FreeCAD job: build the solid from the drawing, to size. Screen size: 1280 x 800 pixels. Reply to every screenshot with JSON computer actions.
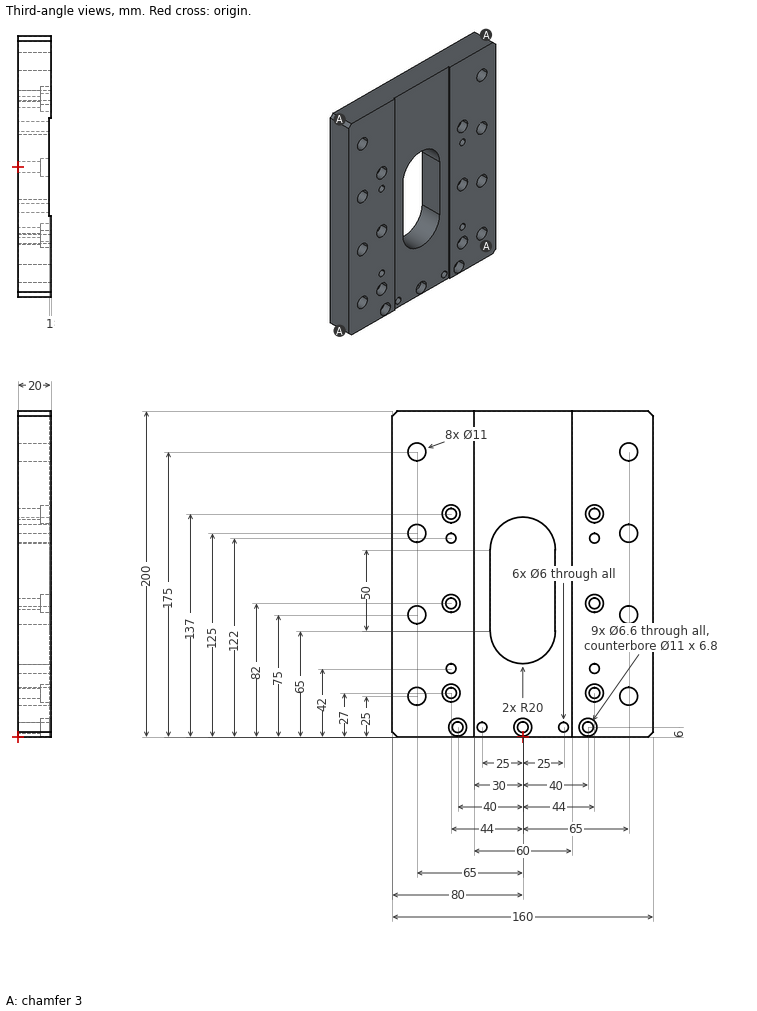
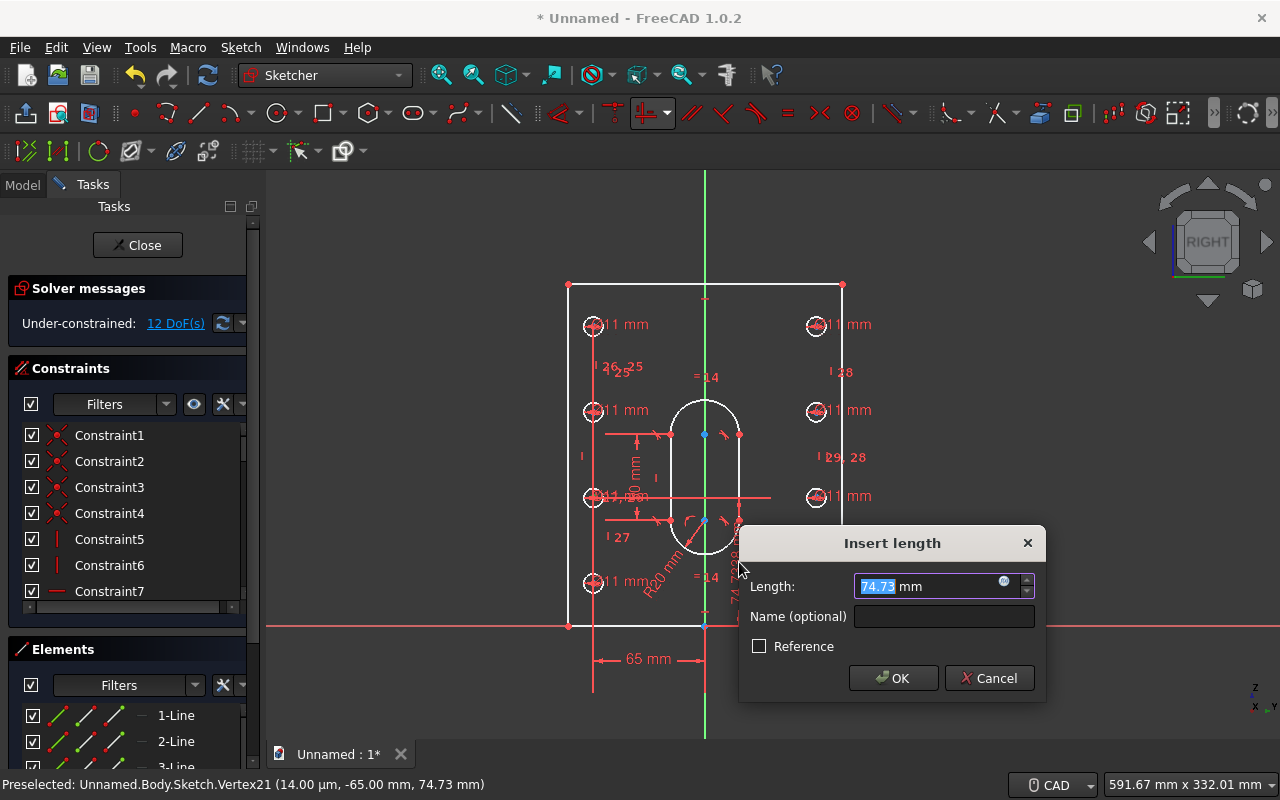
{"action": "type", "text": "75"}
{"action": "key", "text": "Return"}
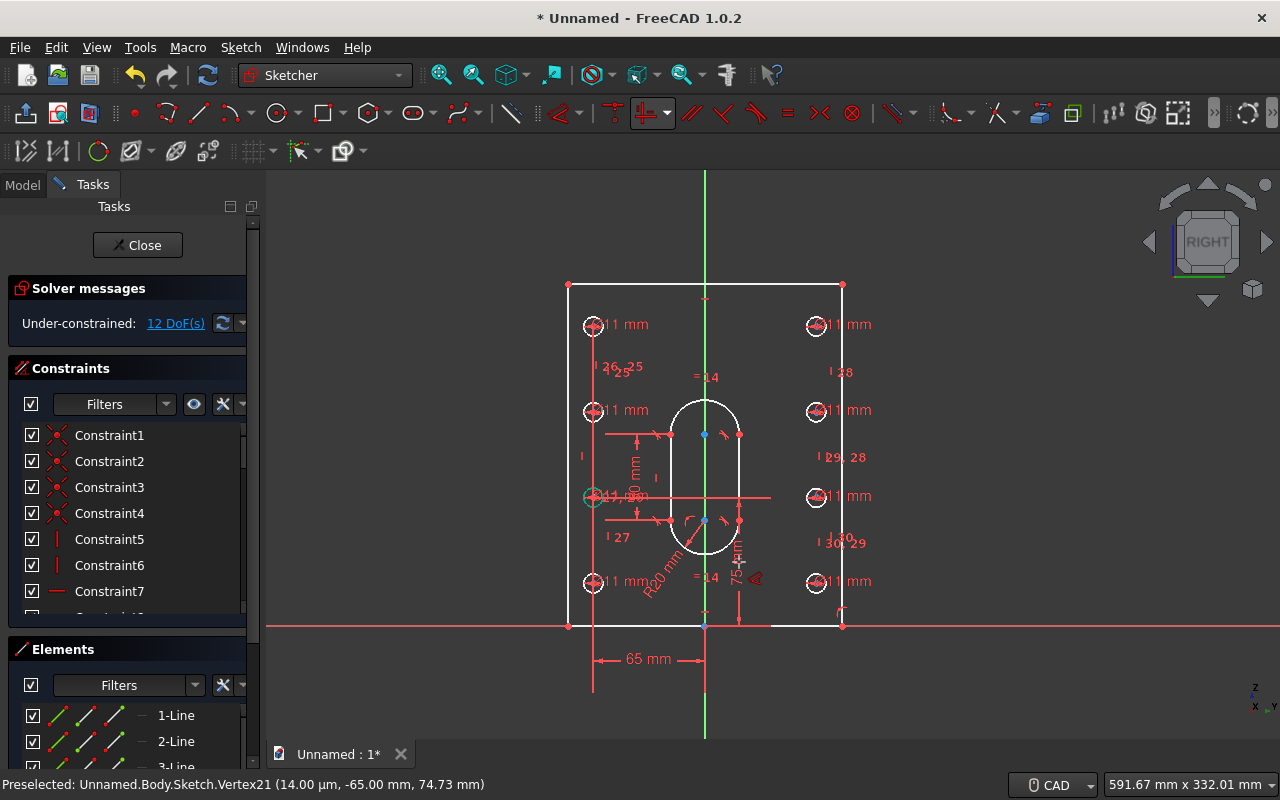
{"action": "left_click", "coordinate": [593, 583]}
{"action": "left_click", "coordinate": [739, 605]}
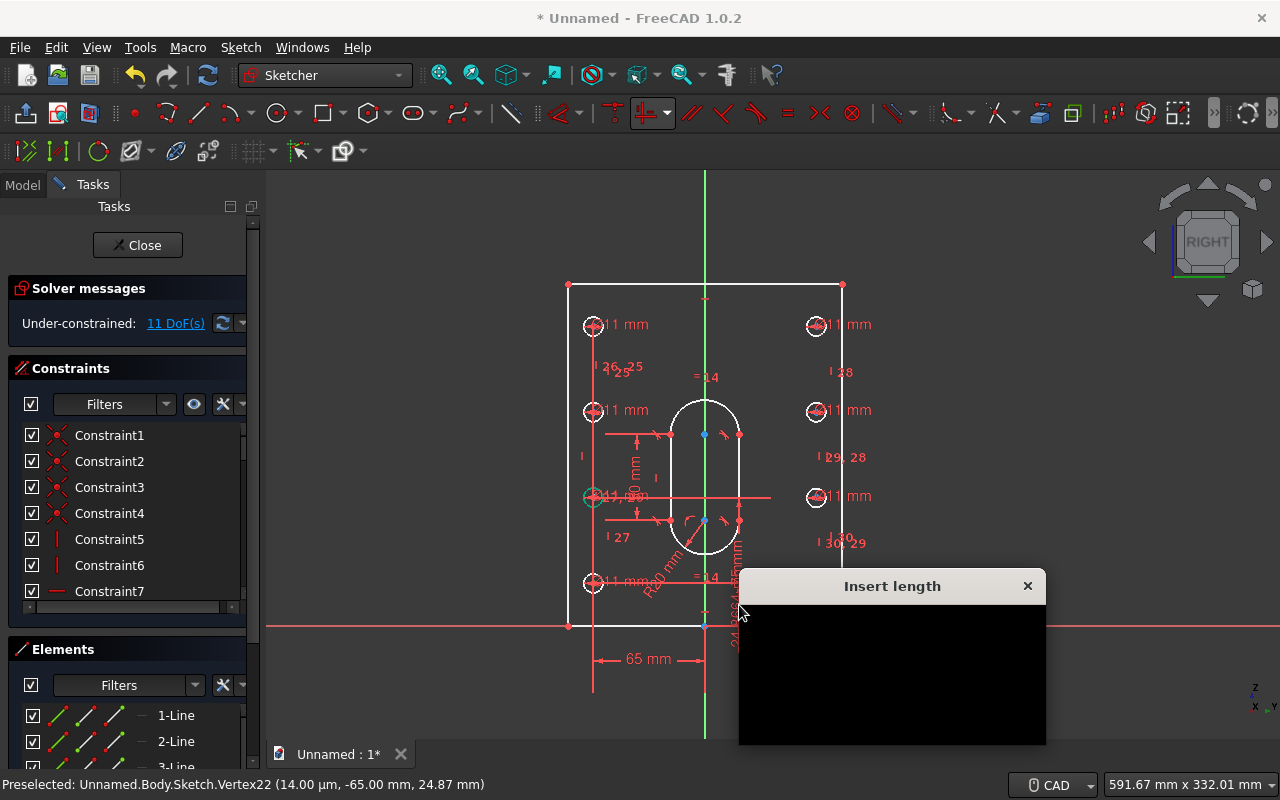
{"action": "type", "text": "25"}
{"action": "key", "text": "Return"}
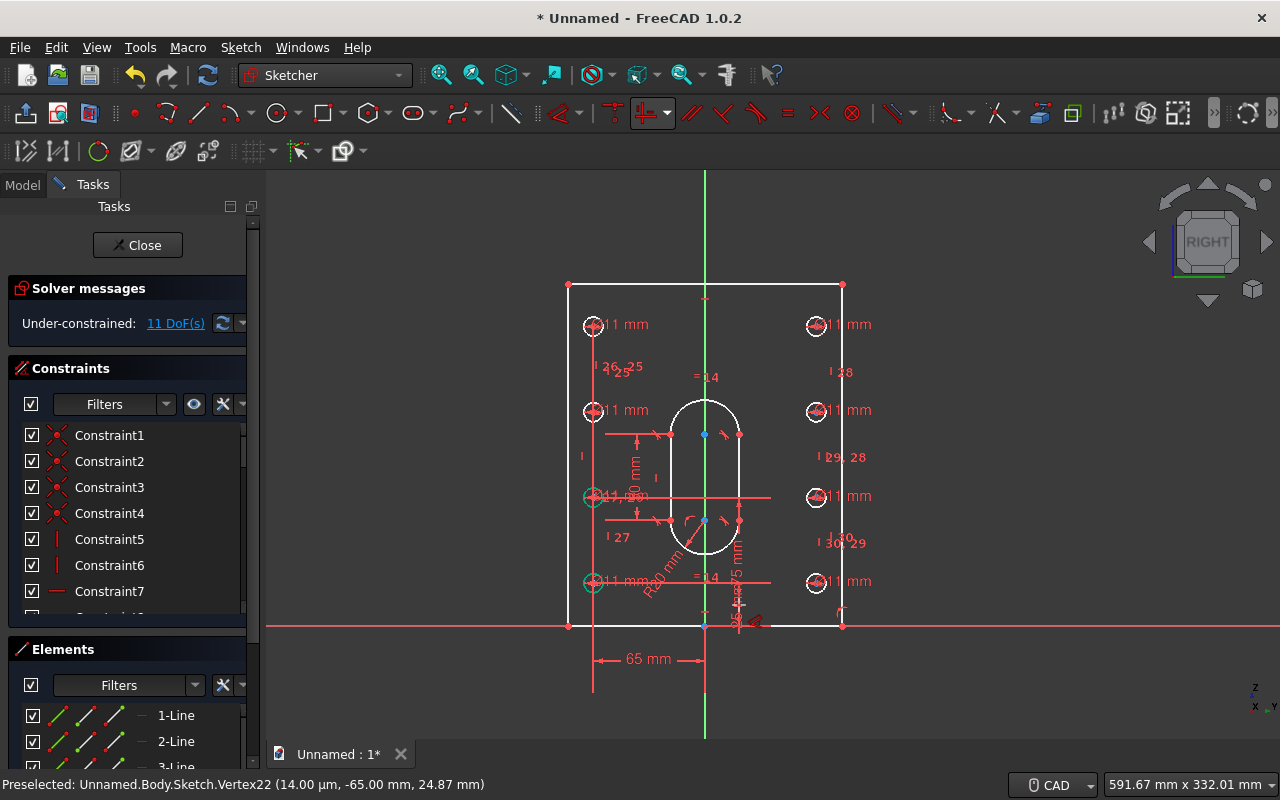
{"action": "left_click", "coordinate": [816, 327]}
{"action": "left_click", "coordinate": [761, 660]}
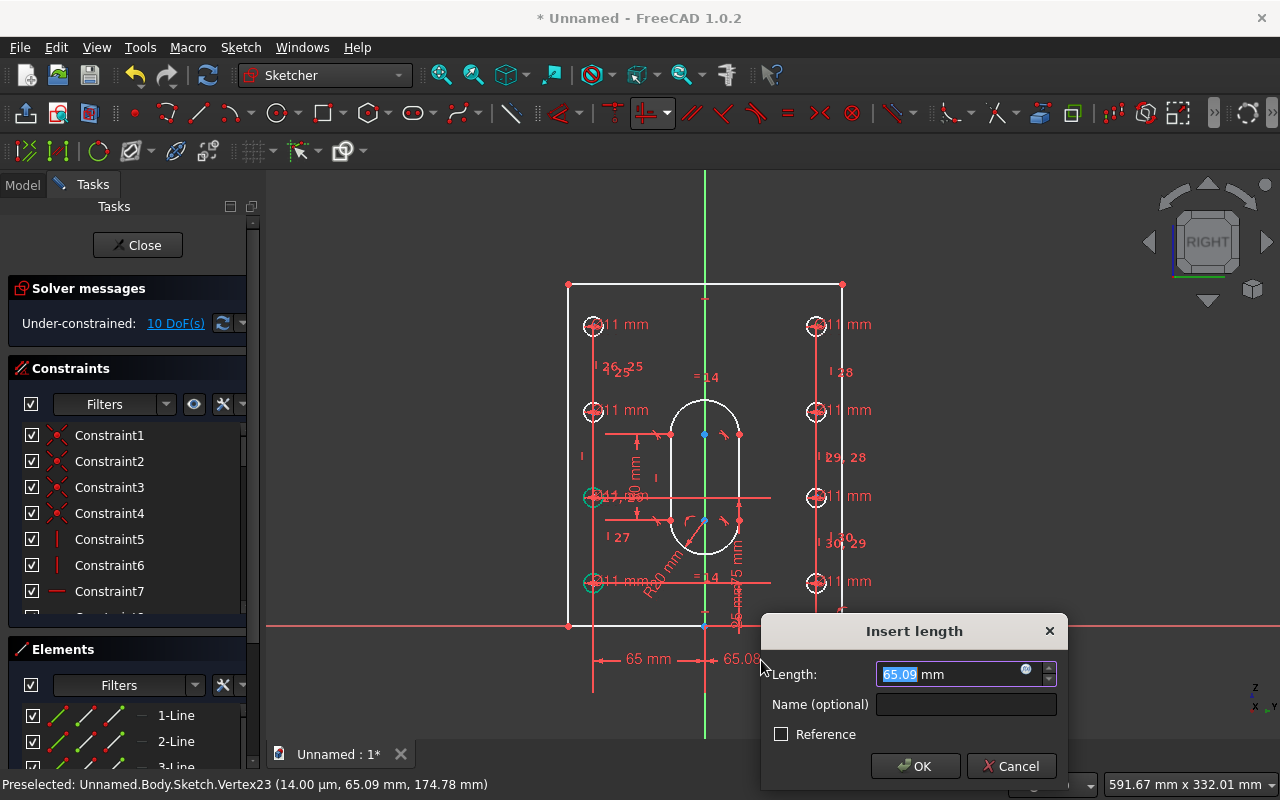
{"action": "type", "text": "65"}
{"action": "key", "text": "Return"}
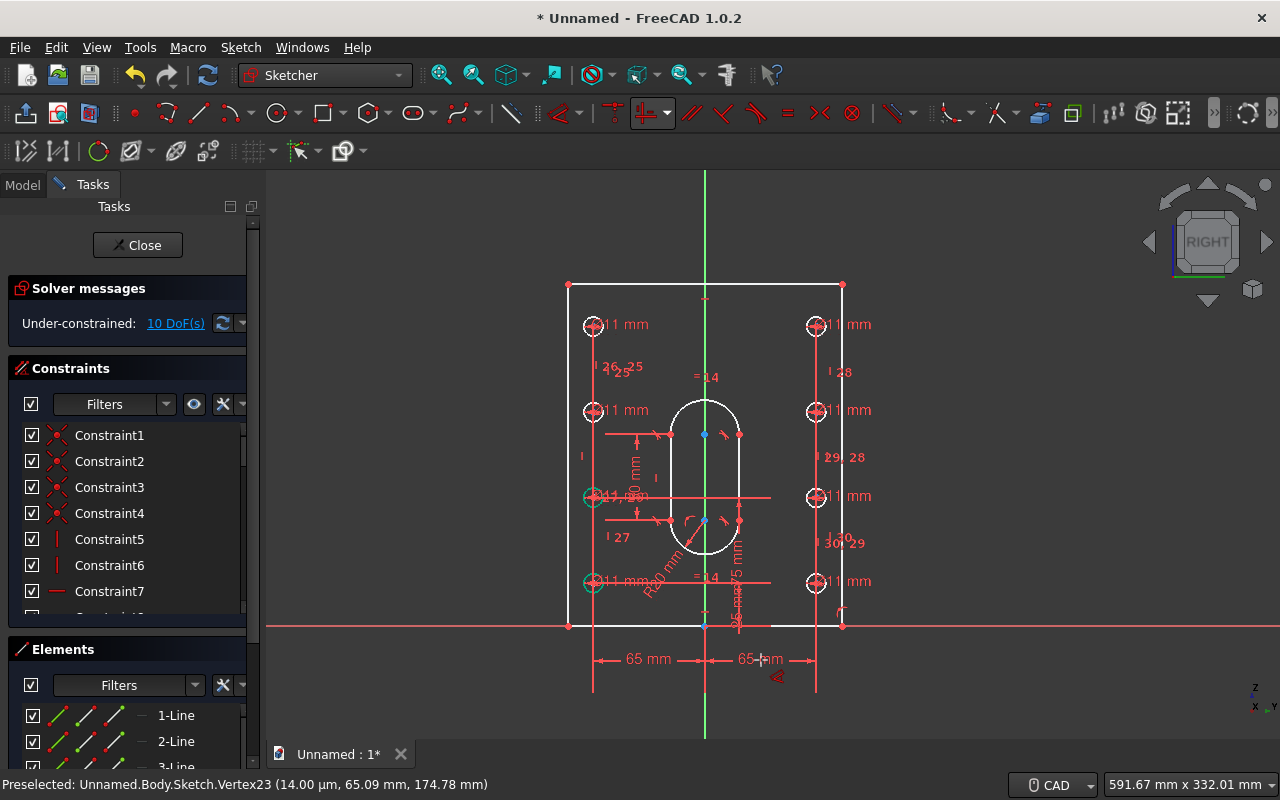
{"action": "left_click", "coordinate": [816, 498]}
{"action": "left_click", "coordinate": [874, 562]}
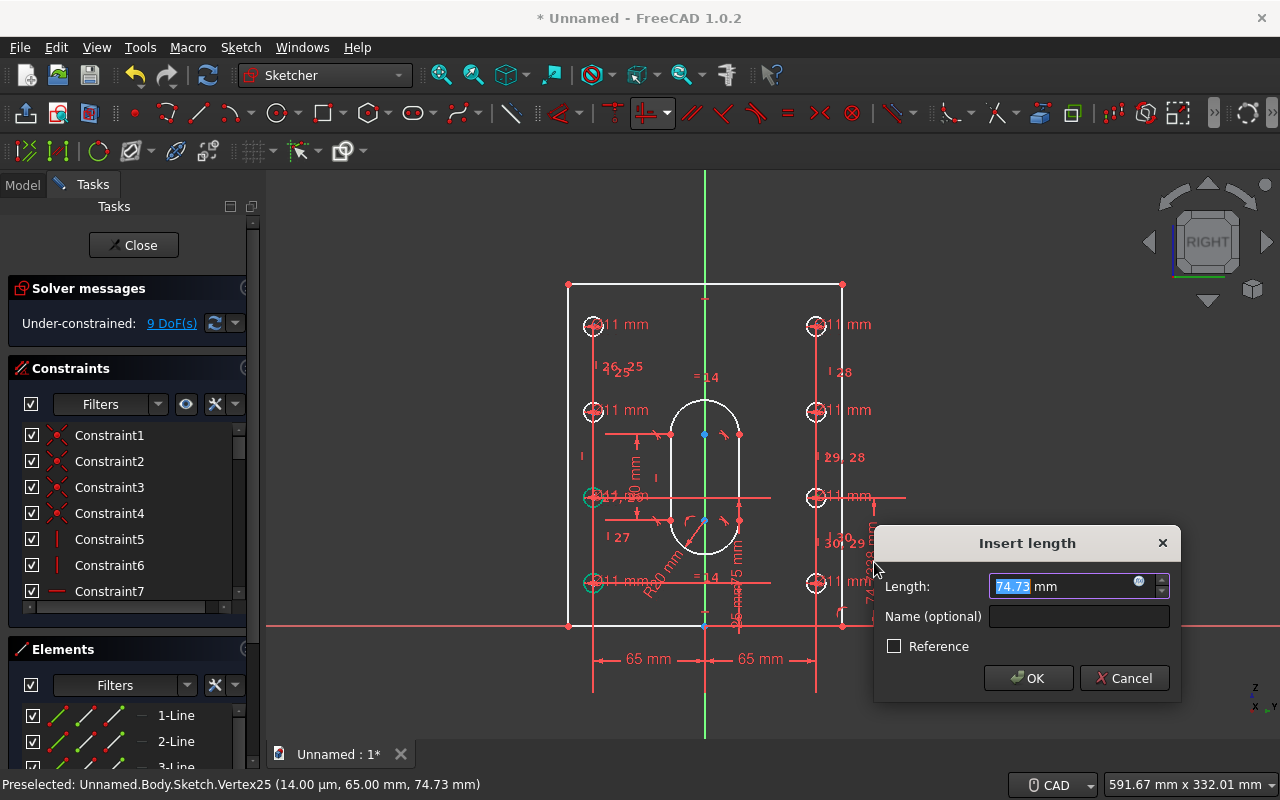
{"action": "type", "text": "75"}
{"action": "key", "text": "Return"}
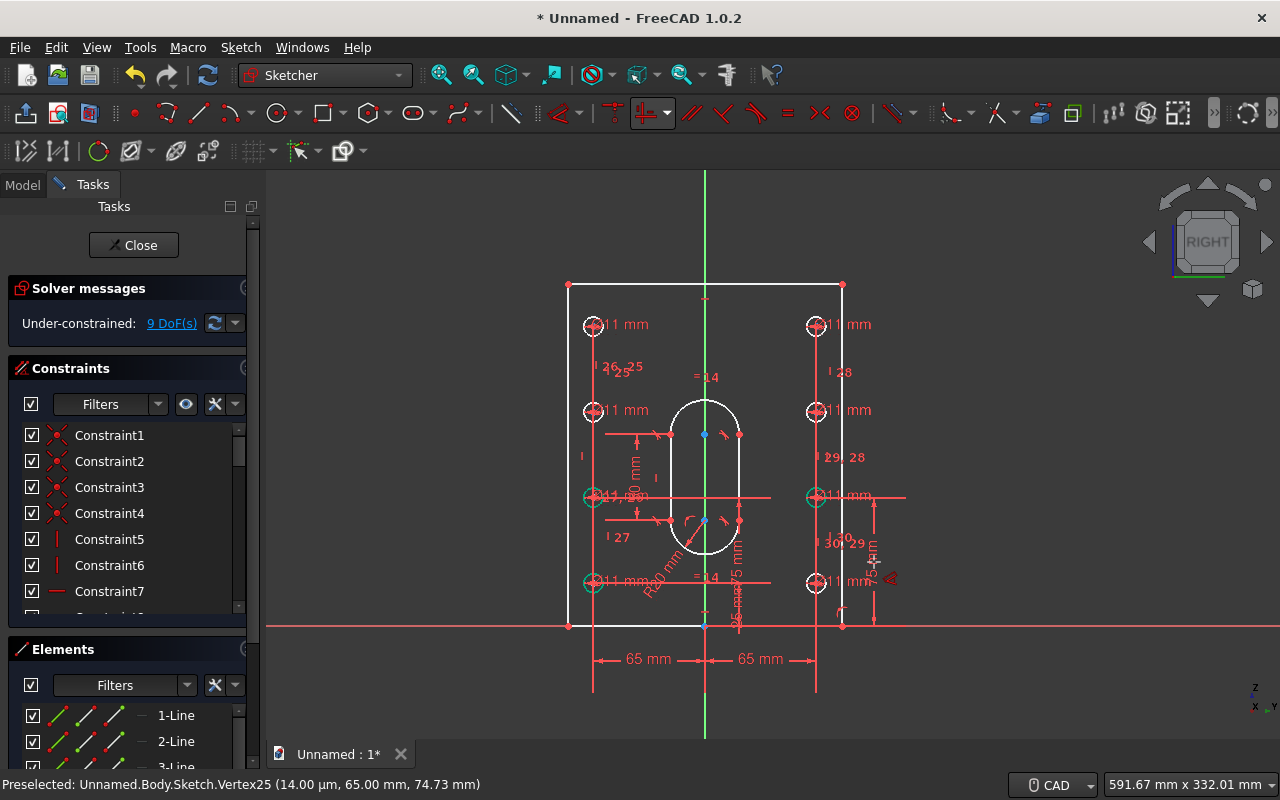
{"action": "left_click", "coordinate": [816, 583]}
{"action": "left_click", "coordinate": [874, 605]}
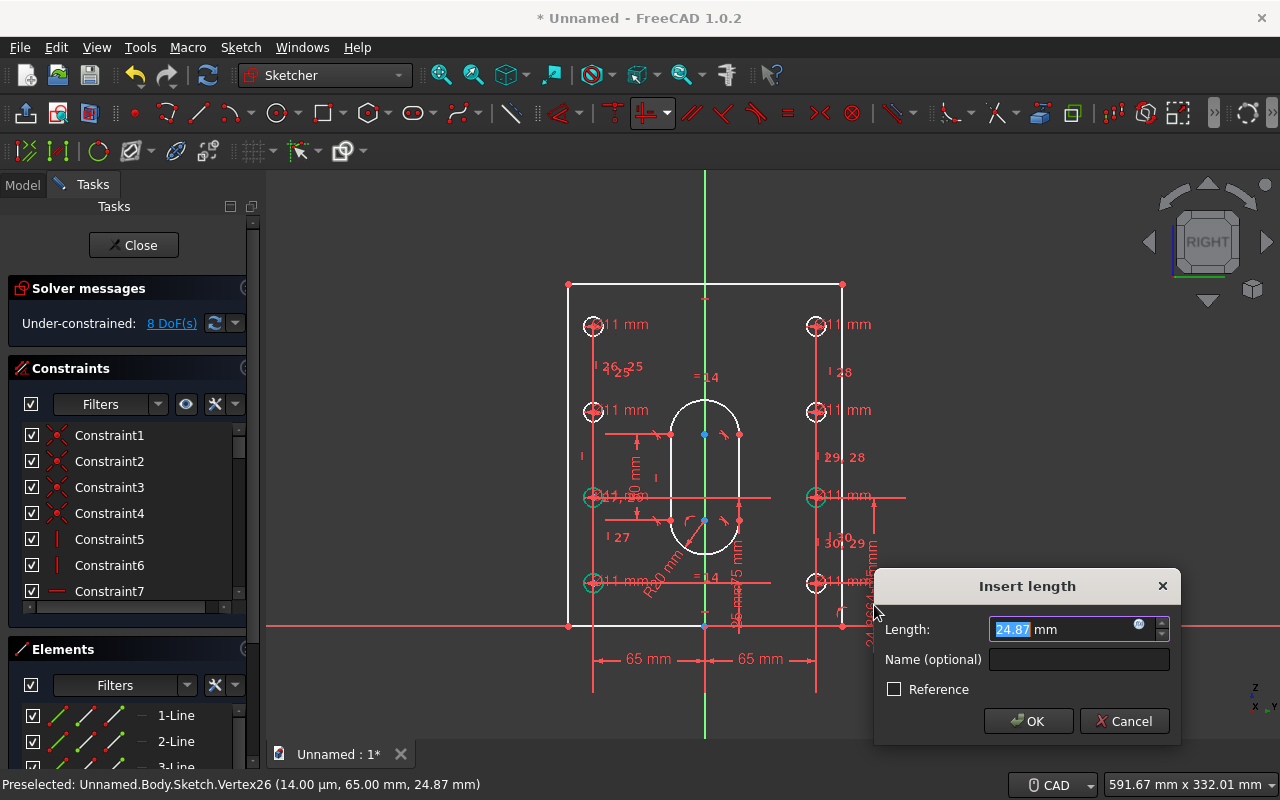
{"action": "type", "text": "25"}
{"action": "key", "text": "Return"}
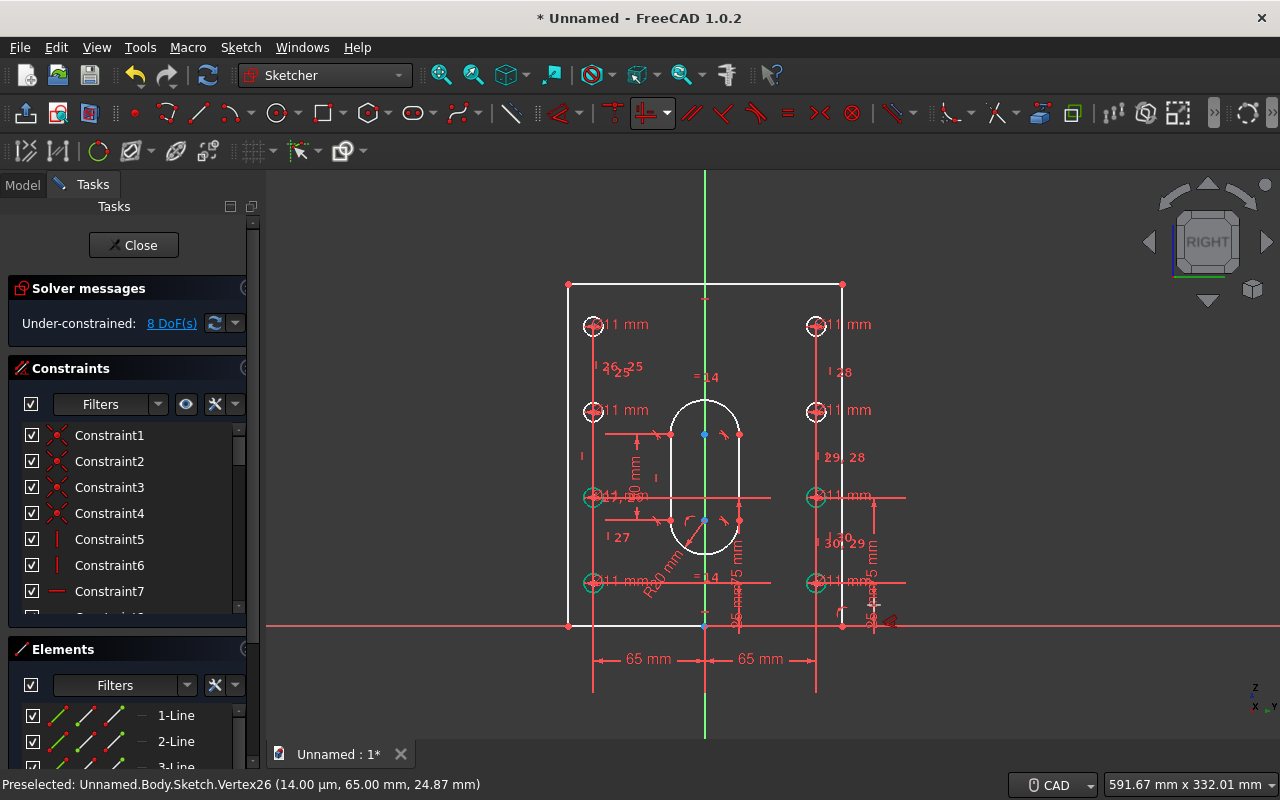
{"action": "left_click", "coordinate": [568, 387]}
{"action": "left_click", "coordinate": [534, 455]}